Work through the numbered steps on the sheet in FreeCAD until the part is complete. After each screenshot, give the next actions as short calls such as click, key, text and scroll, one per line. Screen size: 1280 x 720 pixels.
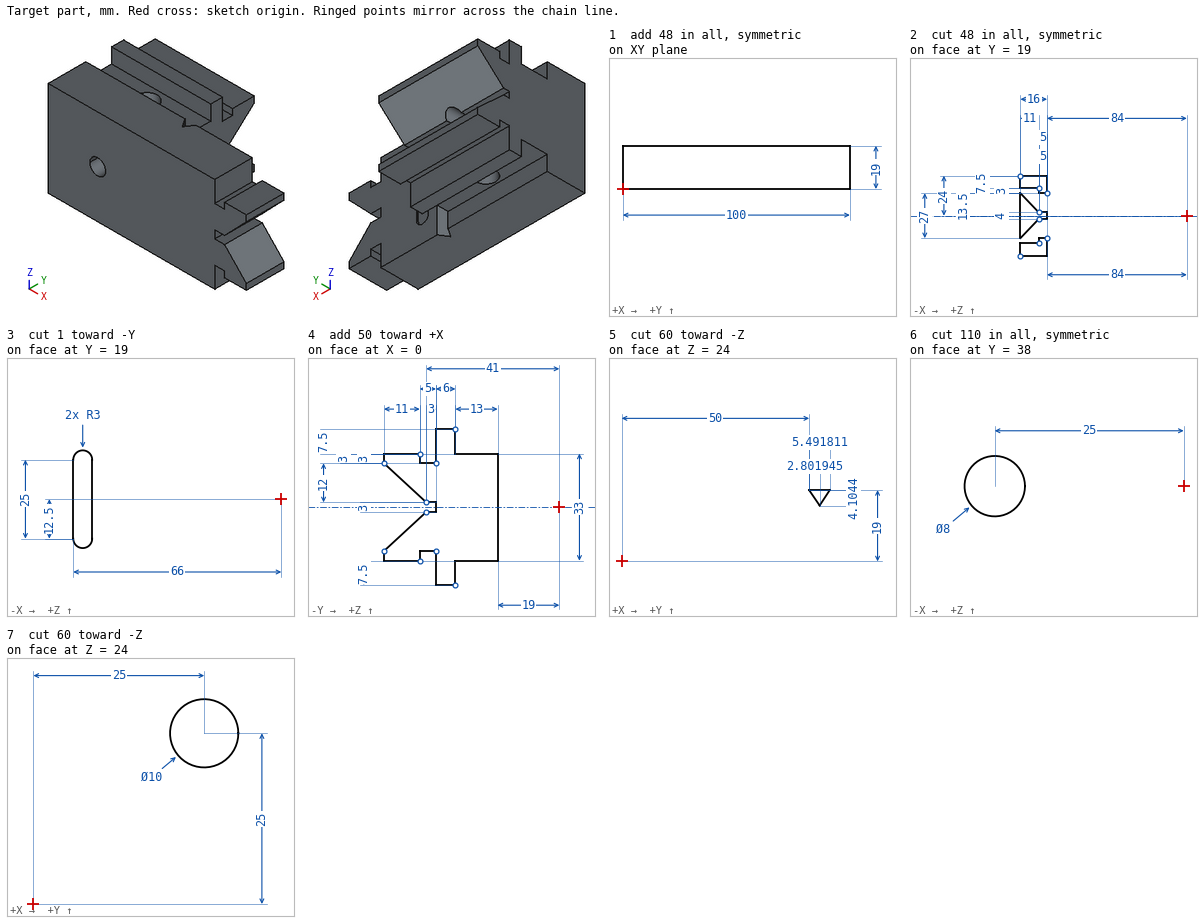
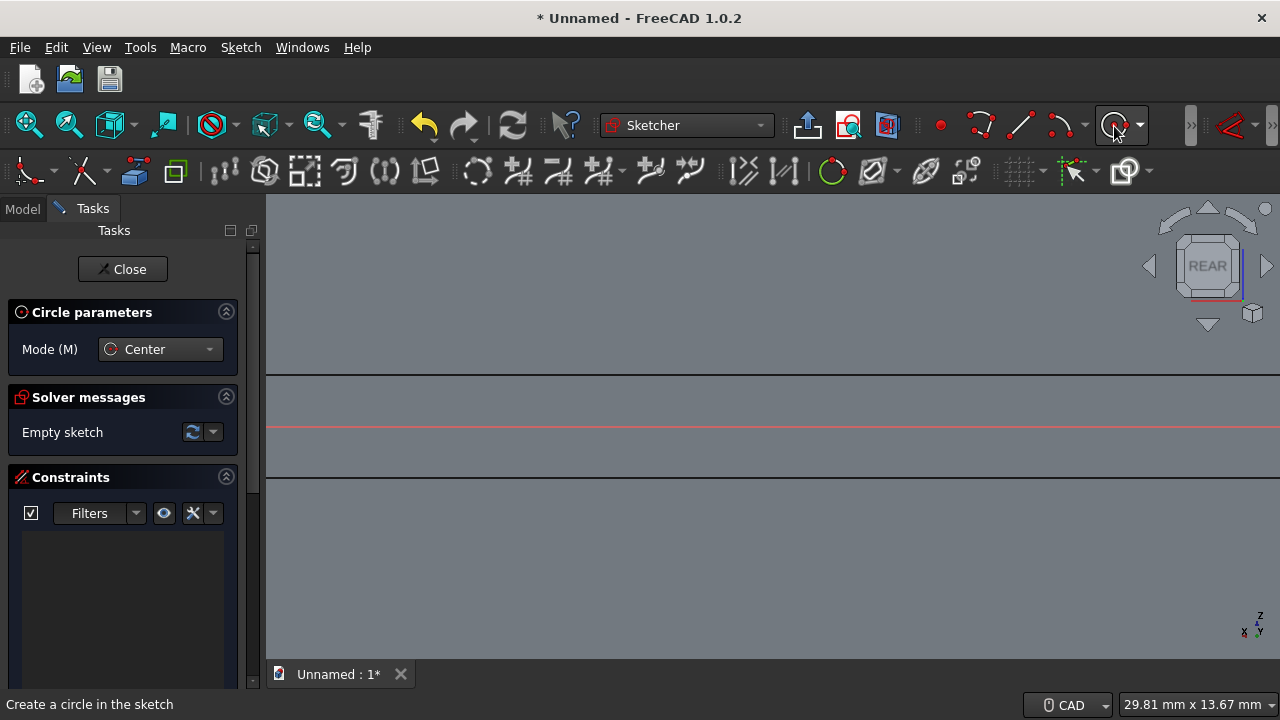
click(696, 426)
click(792, 330)
key(Escape)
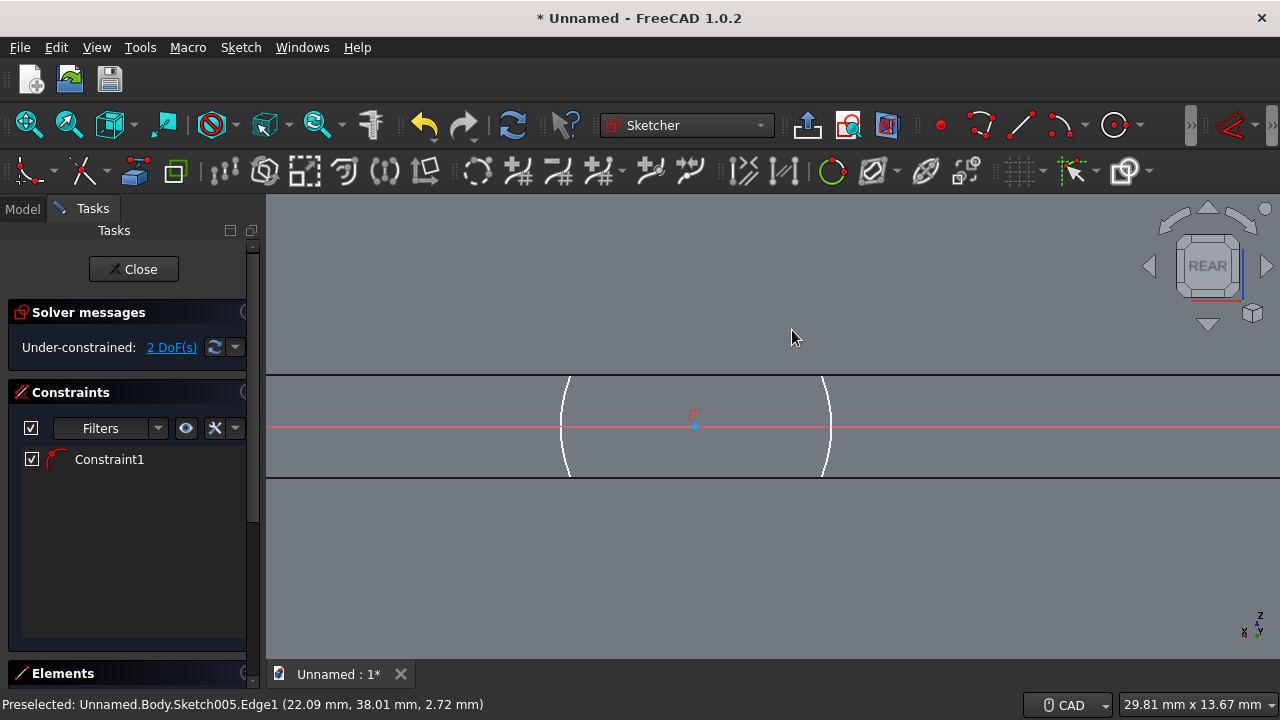
click(1230, 126)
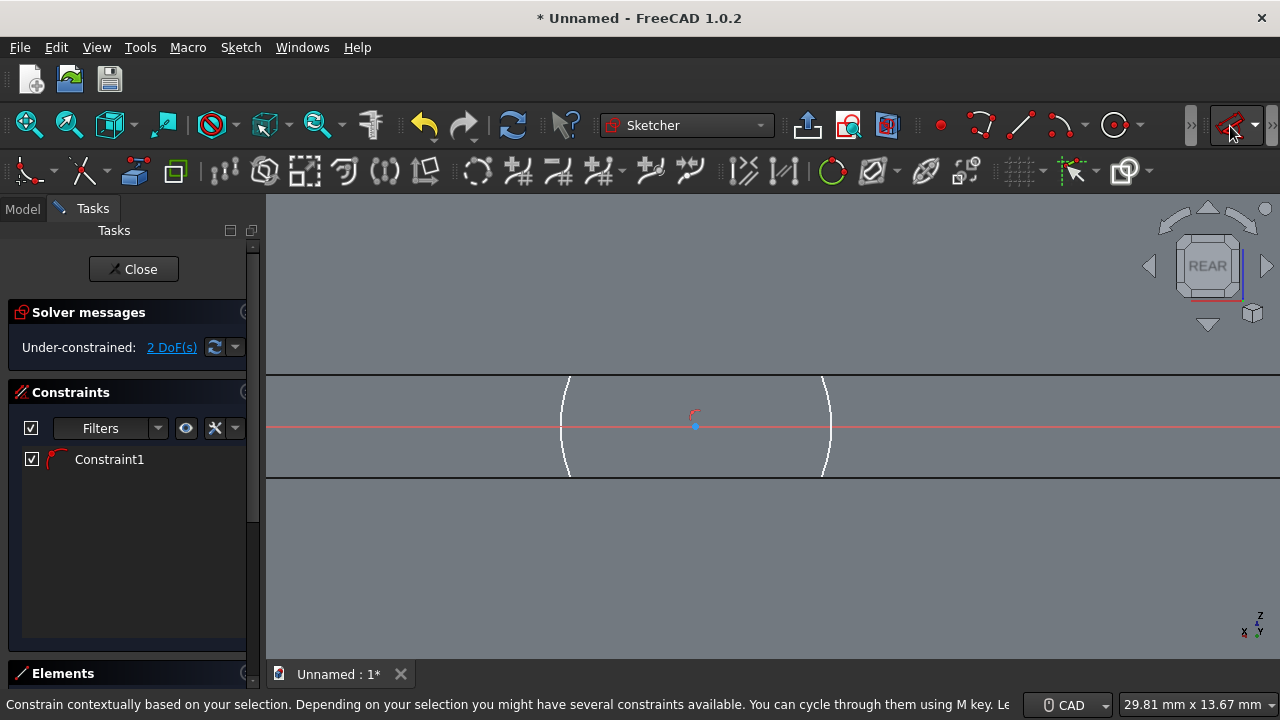
click(791, 330)
click(813, 307)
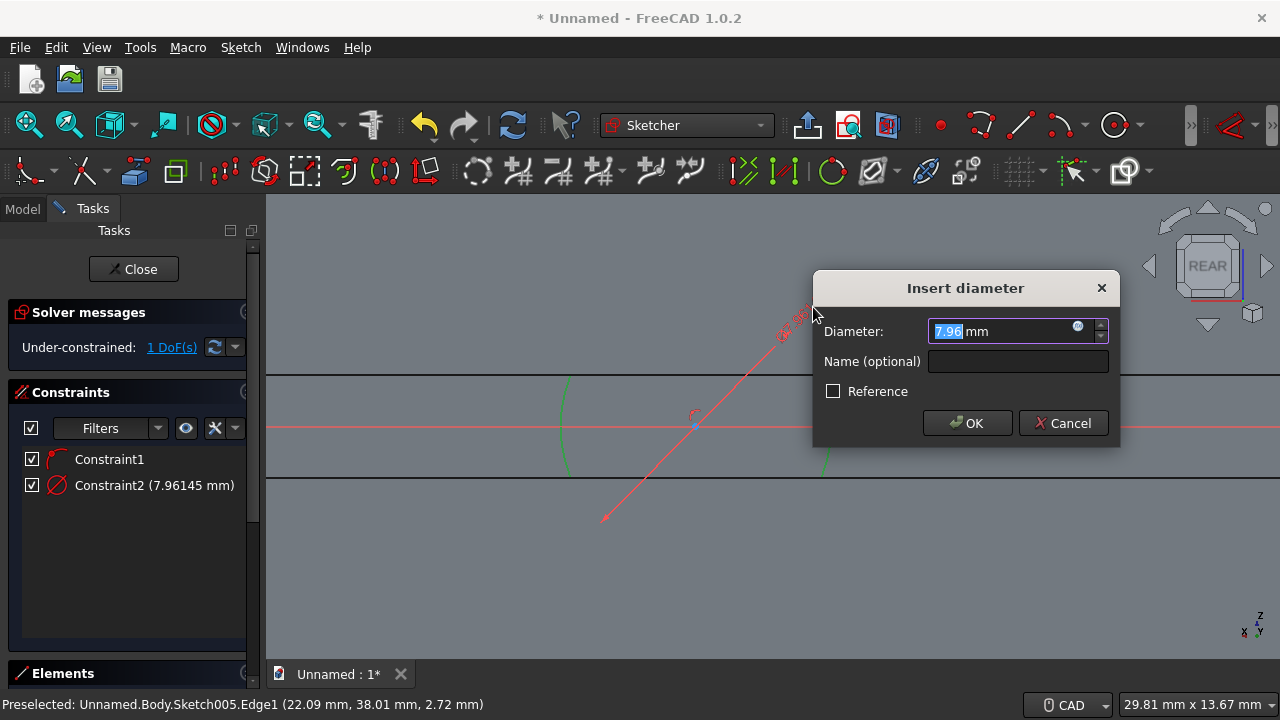
text(8)
key(Return)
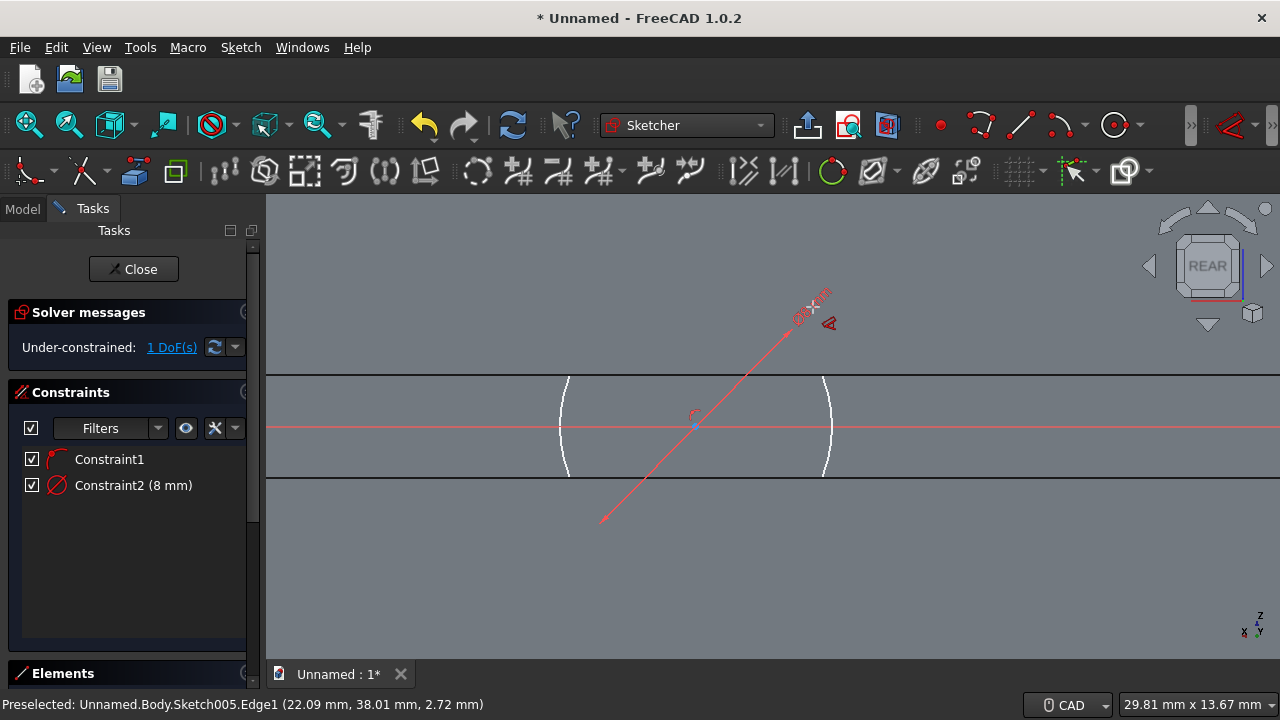
click(696, 426)
click(906, 460)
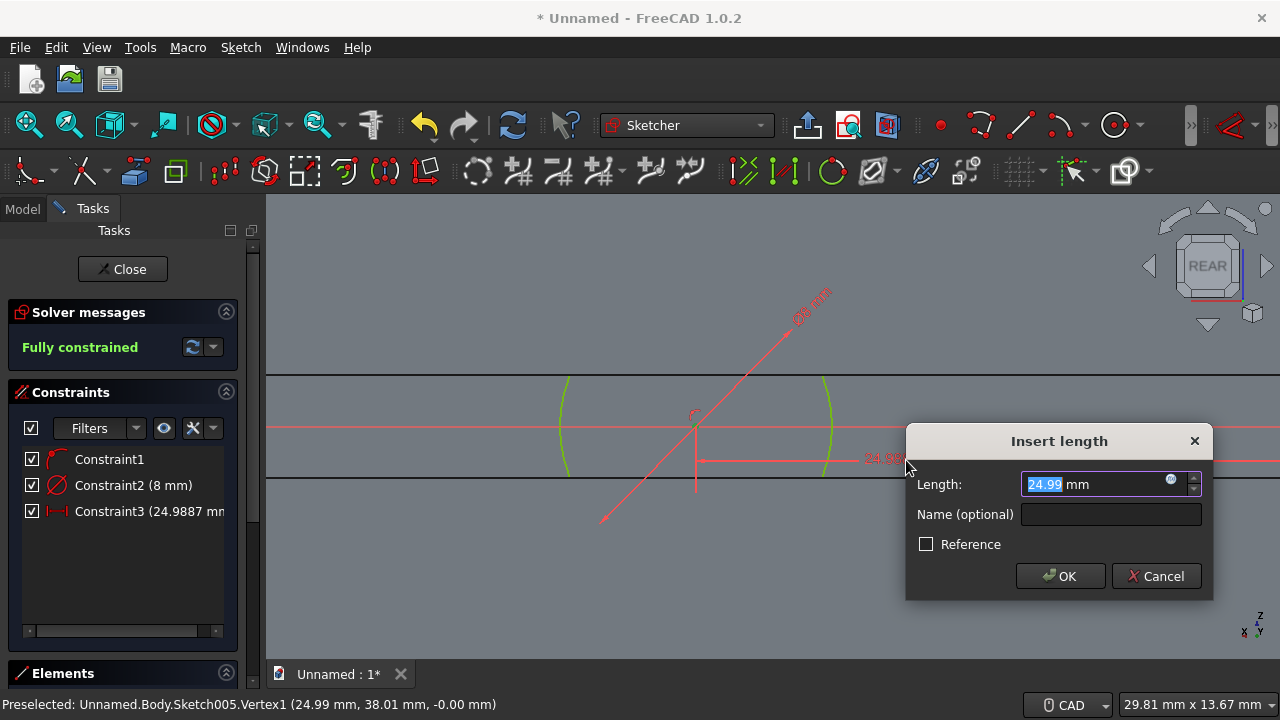
text(25)
key(Return)
key(Escape)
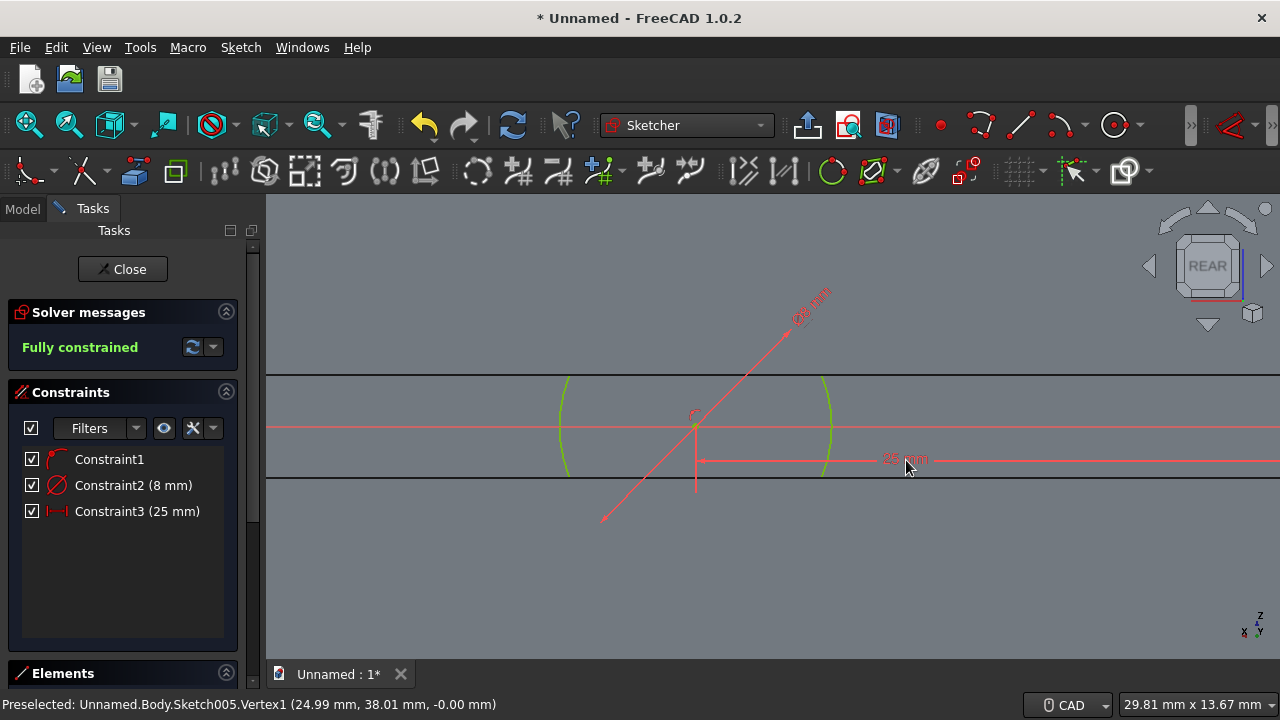
click(123, 269)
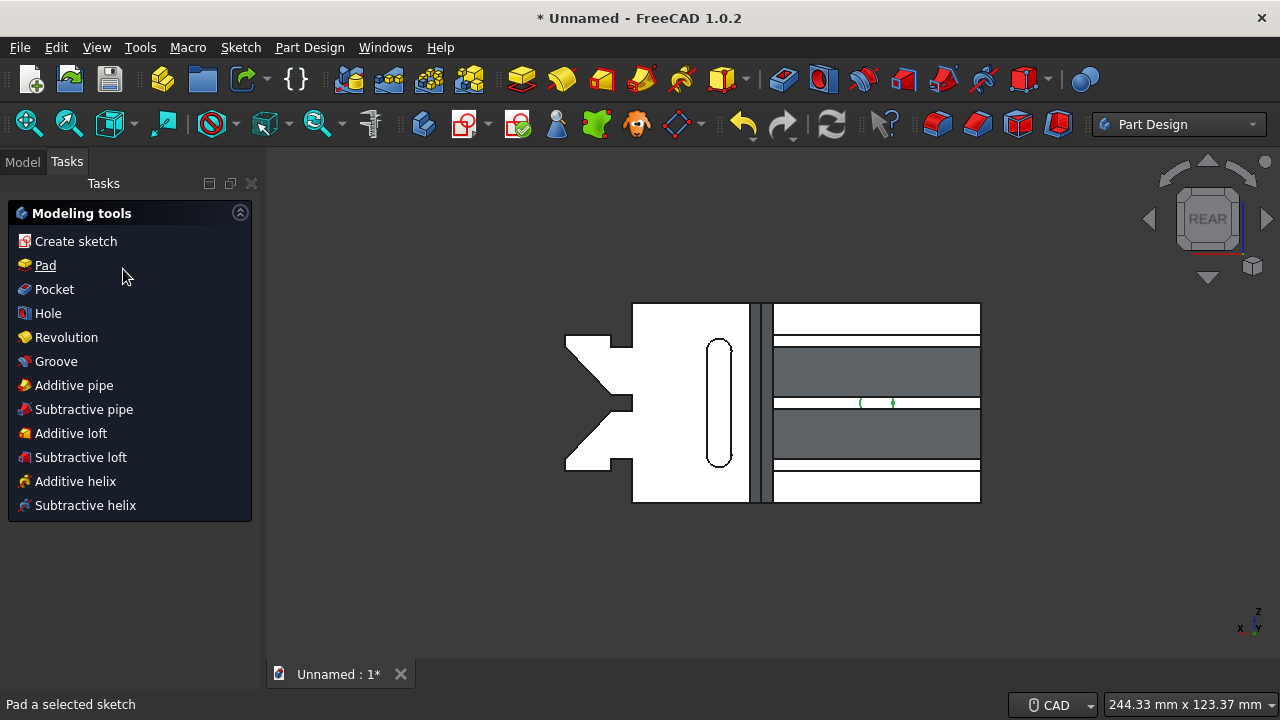
click(784, 80)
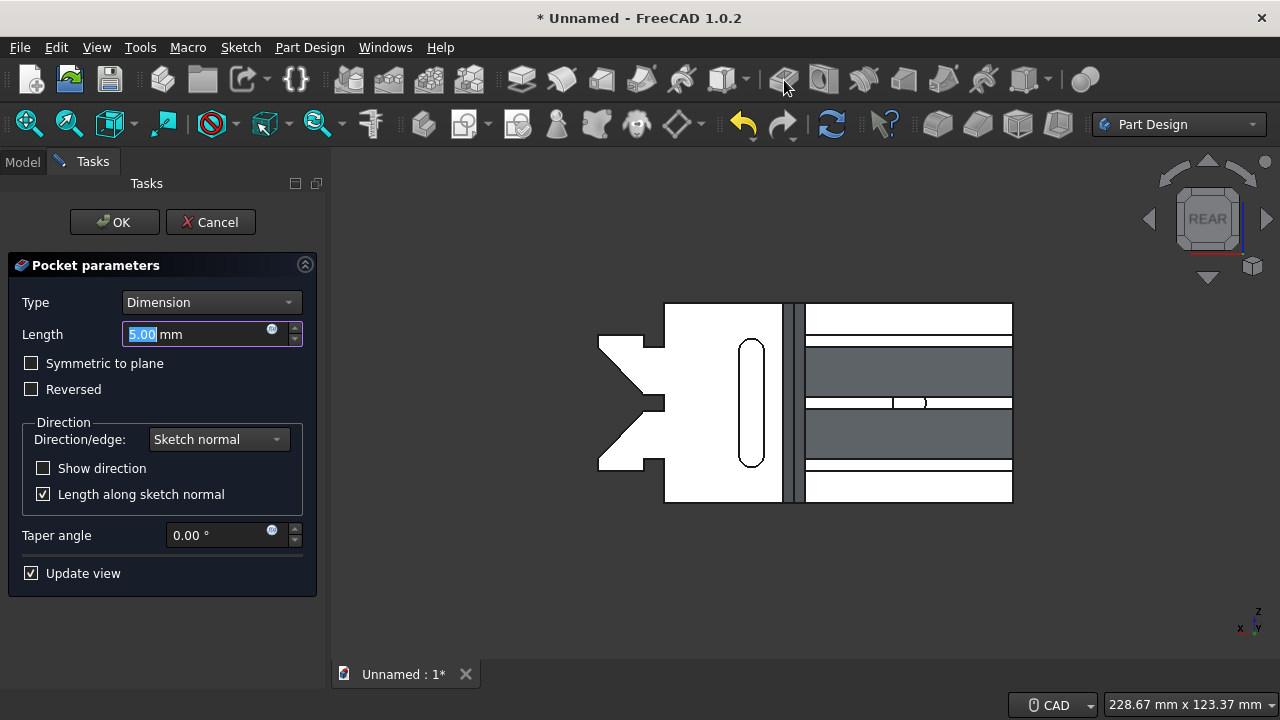
text(110)
key(Tab)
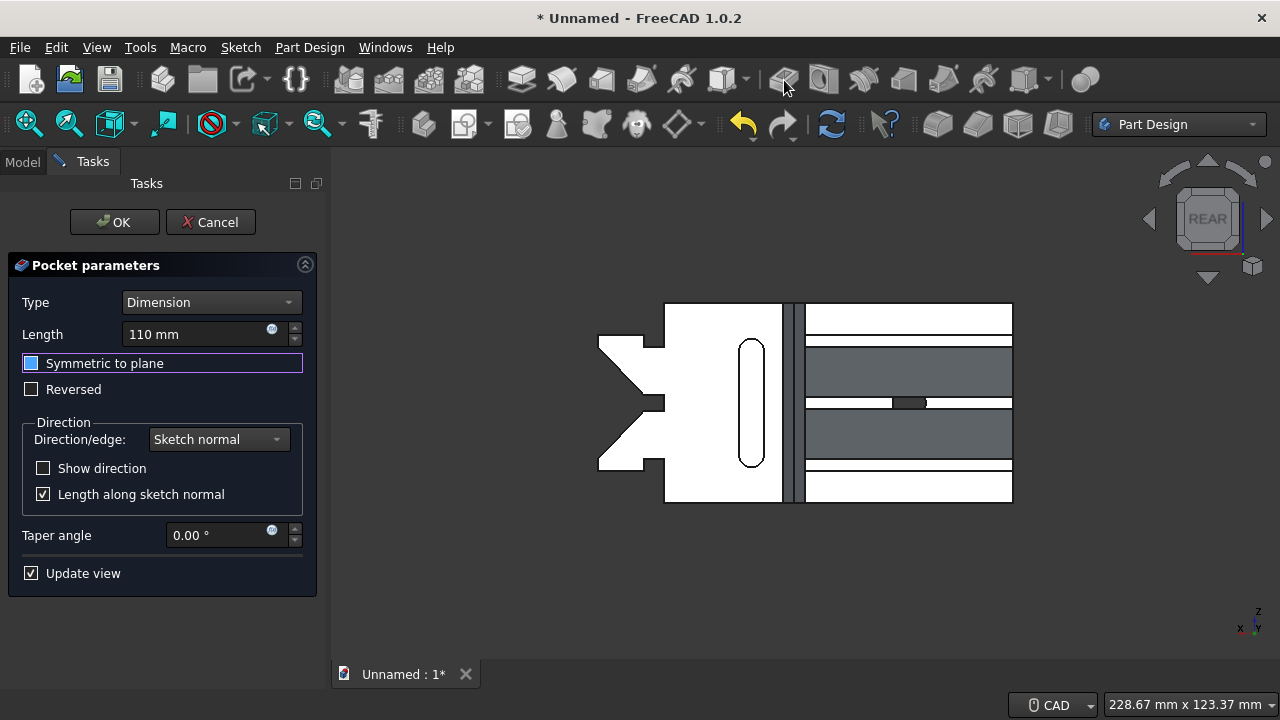
click(30, 363)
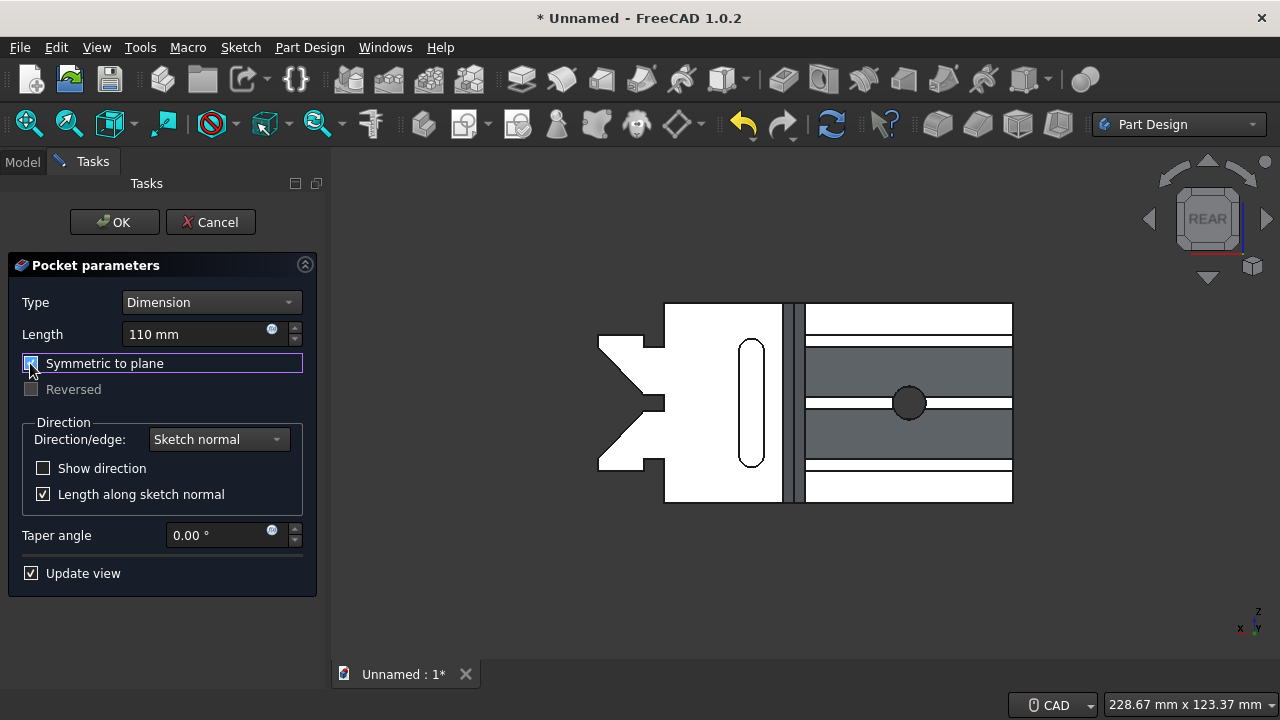
click(115, 222)